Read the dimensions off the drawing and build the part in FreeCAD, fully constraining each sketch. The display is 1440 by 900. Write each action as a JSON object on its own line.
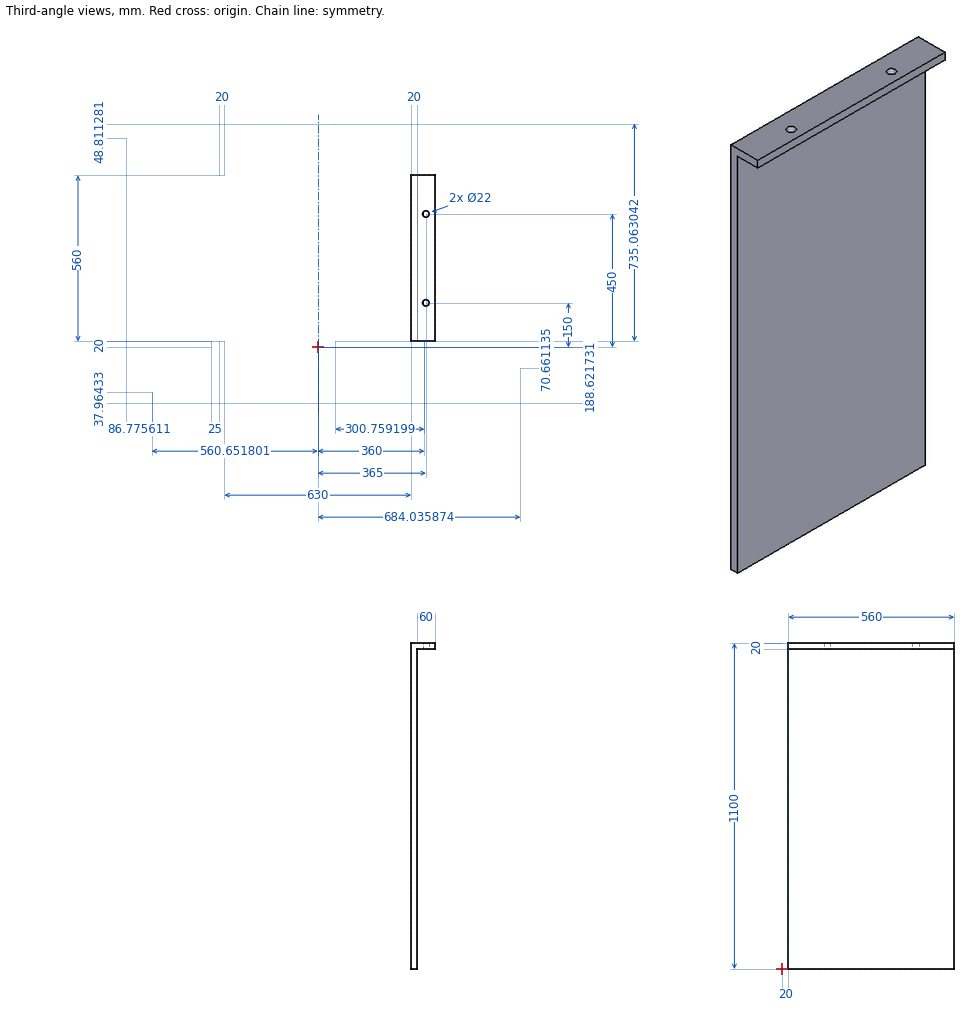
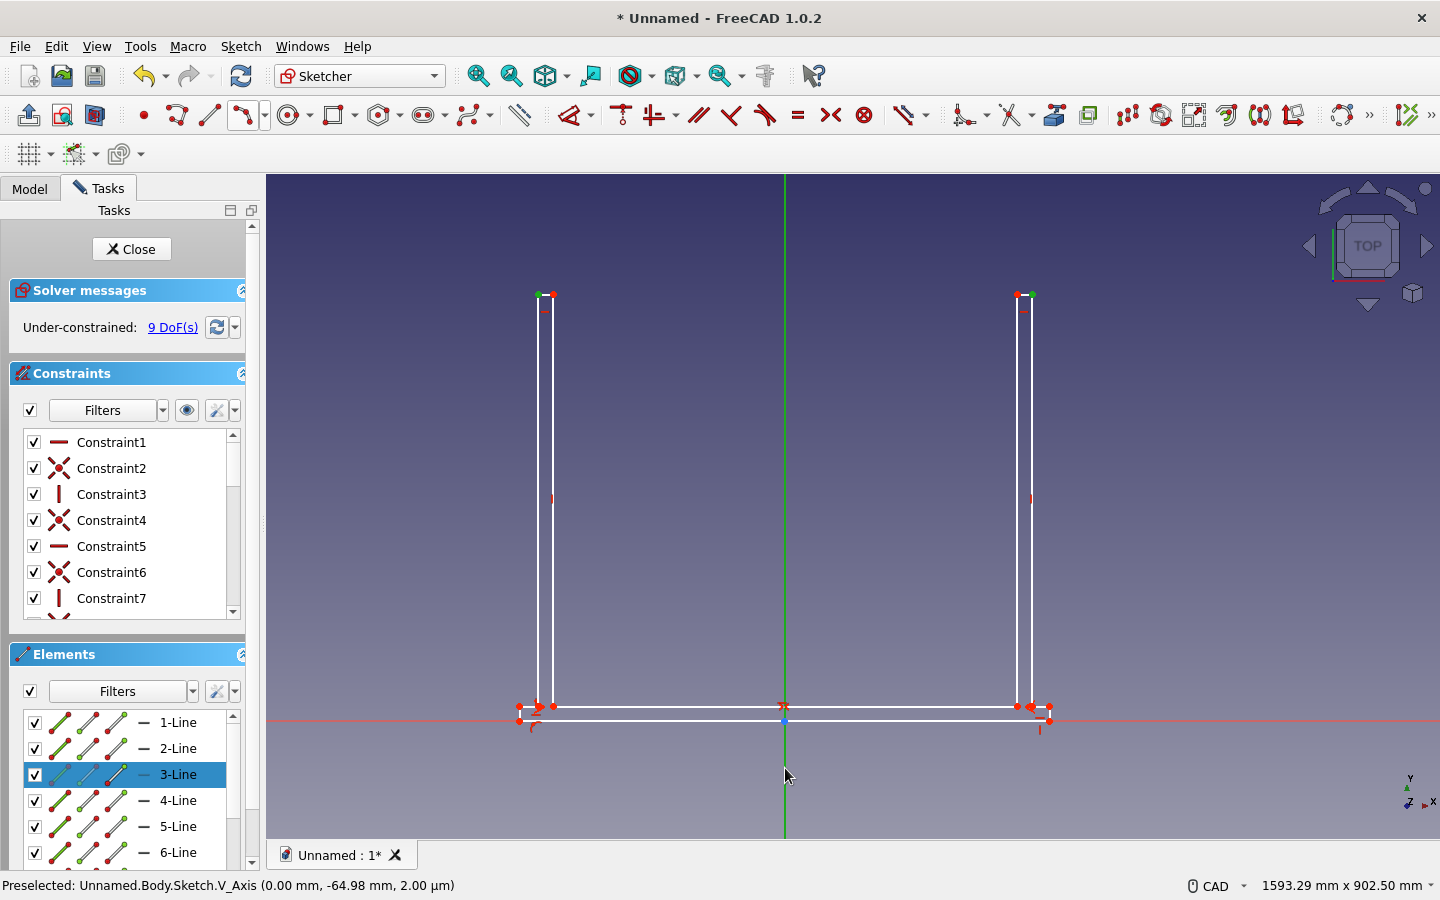
{"action": "key", "text": "s"}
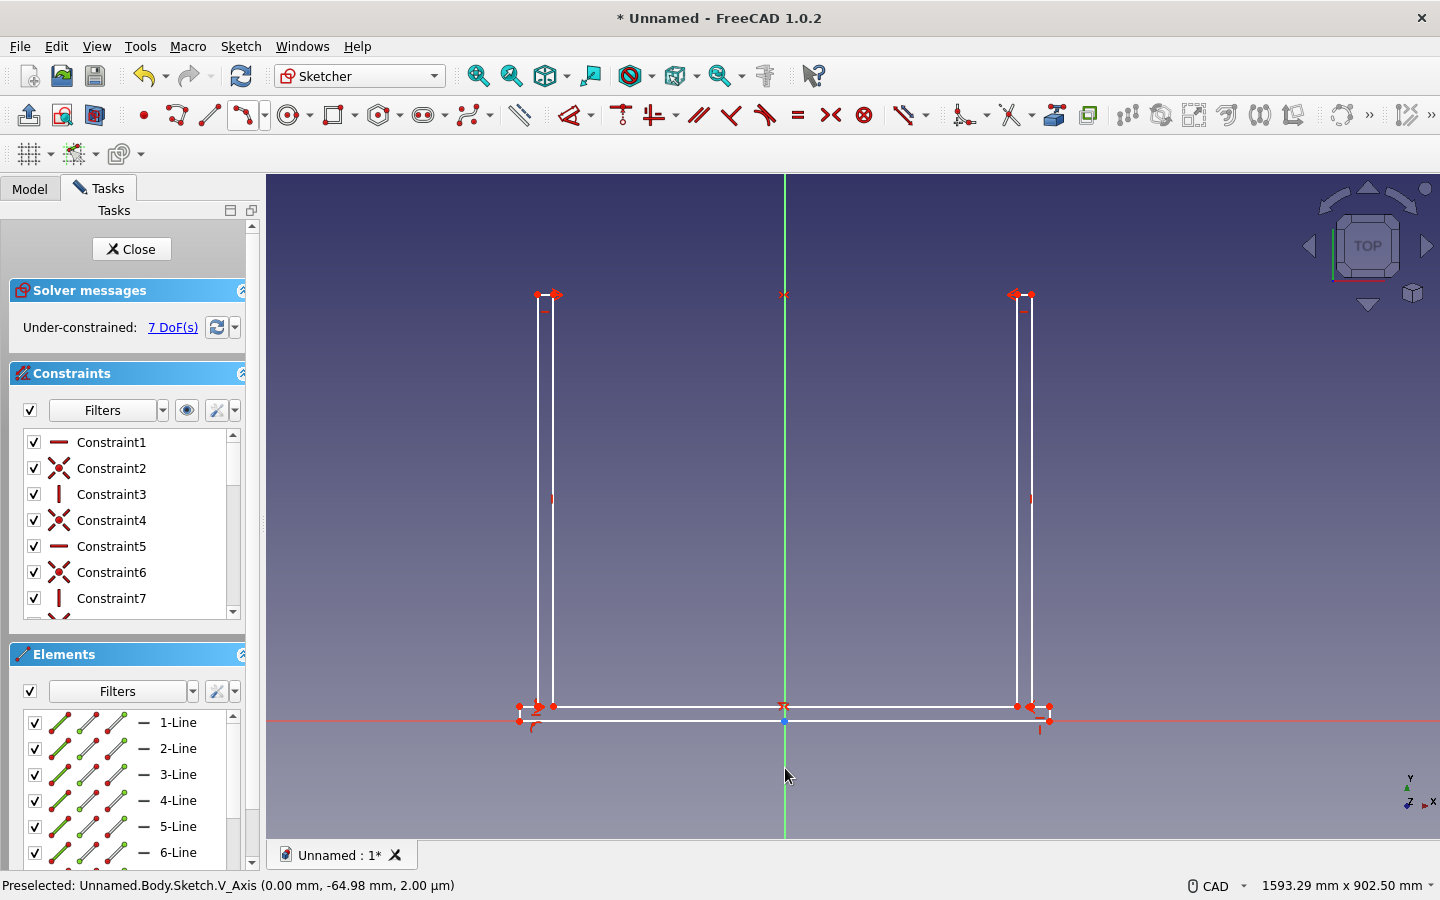
{"action": "left_click", "coordinate": [568, 116]}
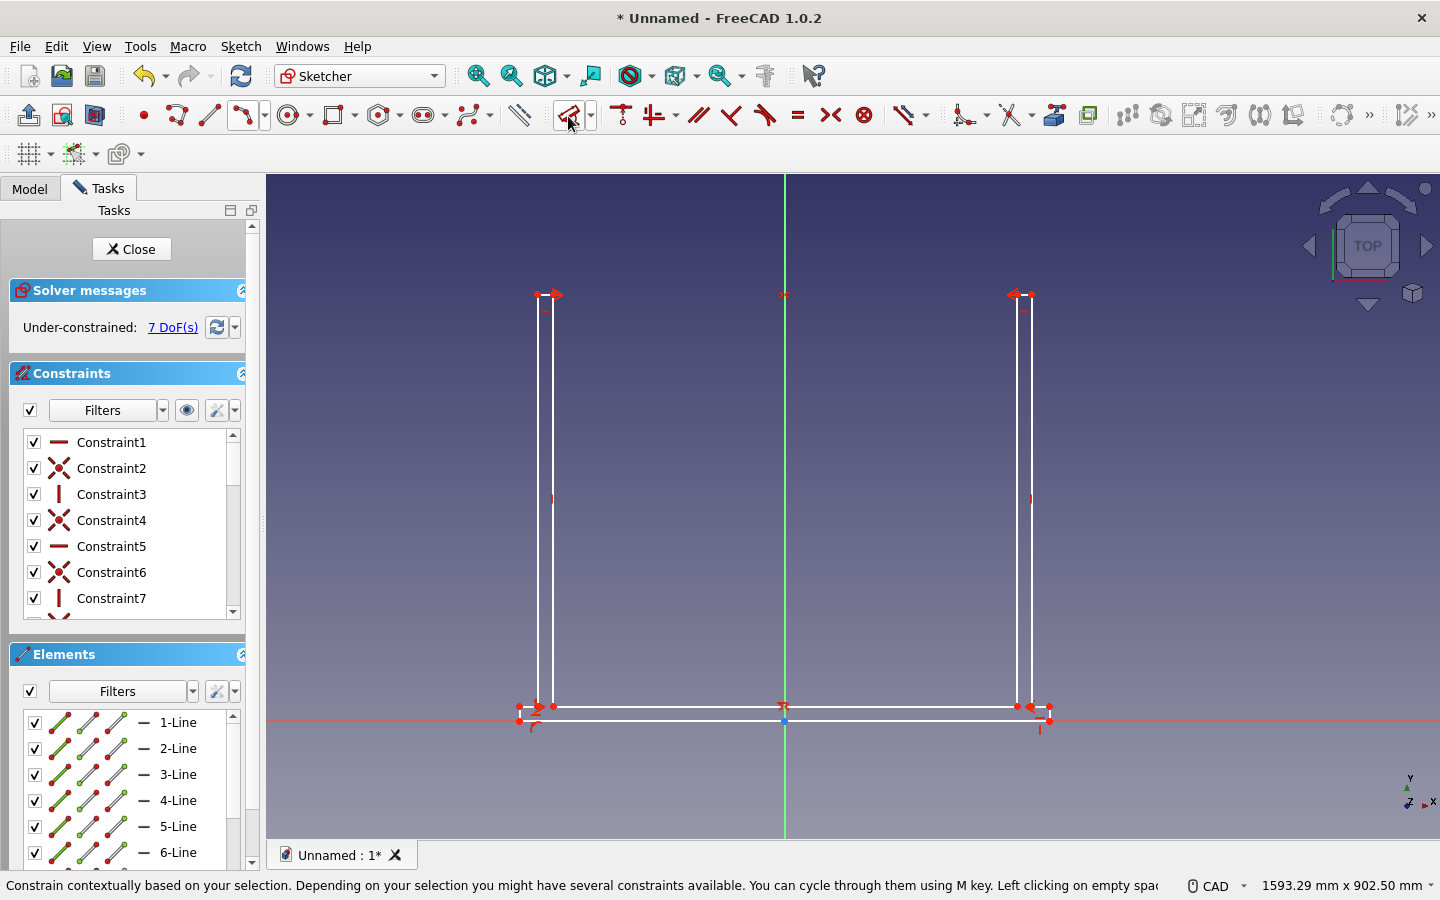
{"action": "scroll", "coordinate": [545, 295], "scroll_direction": "up", "scroll_amount": 5}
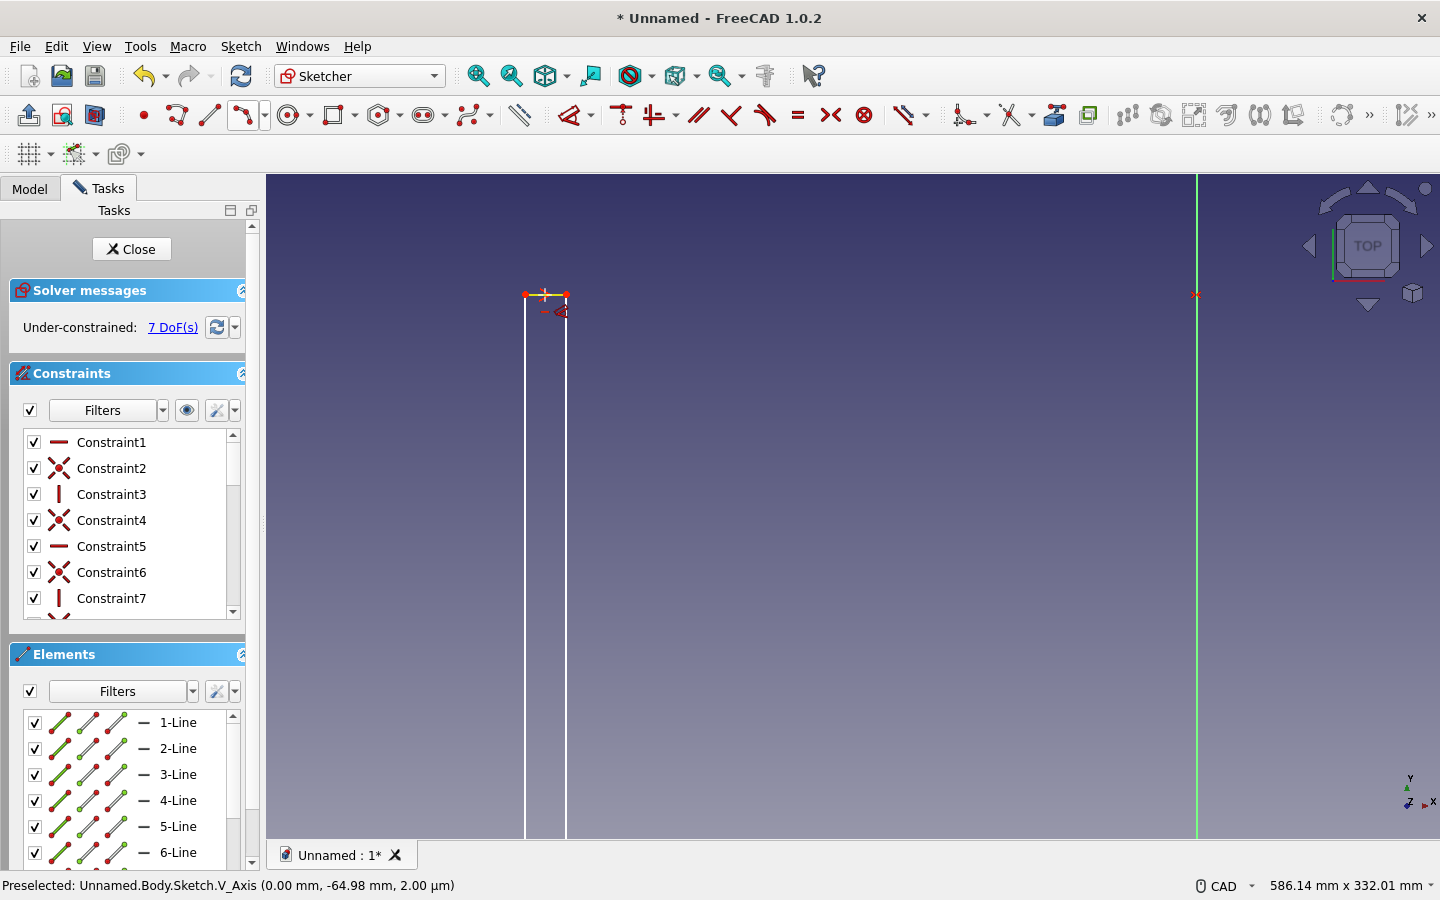
{"action": "left_click", "coordinate": [546, 295]}
{"action": "left_click", "coordinate": [546, 261]}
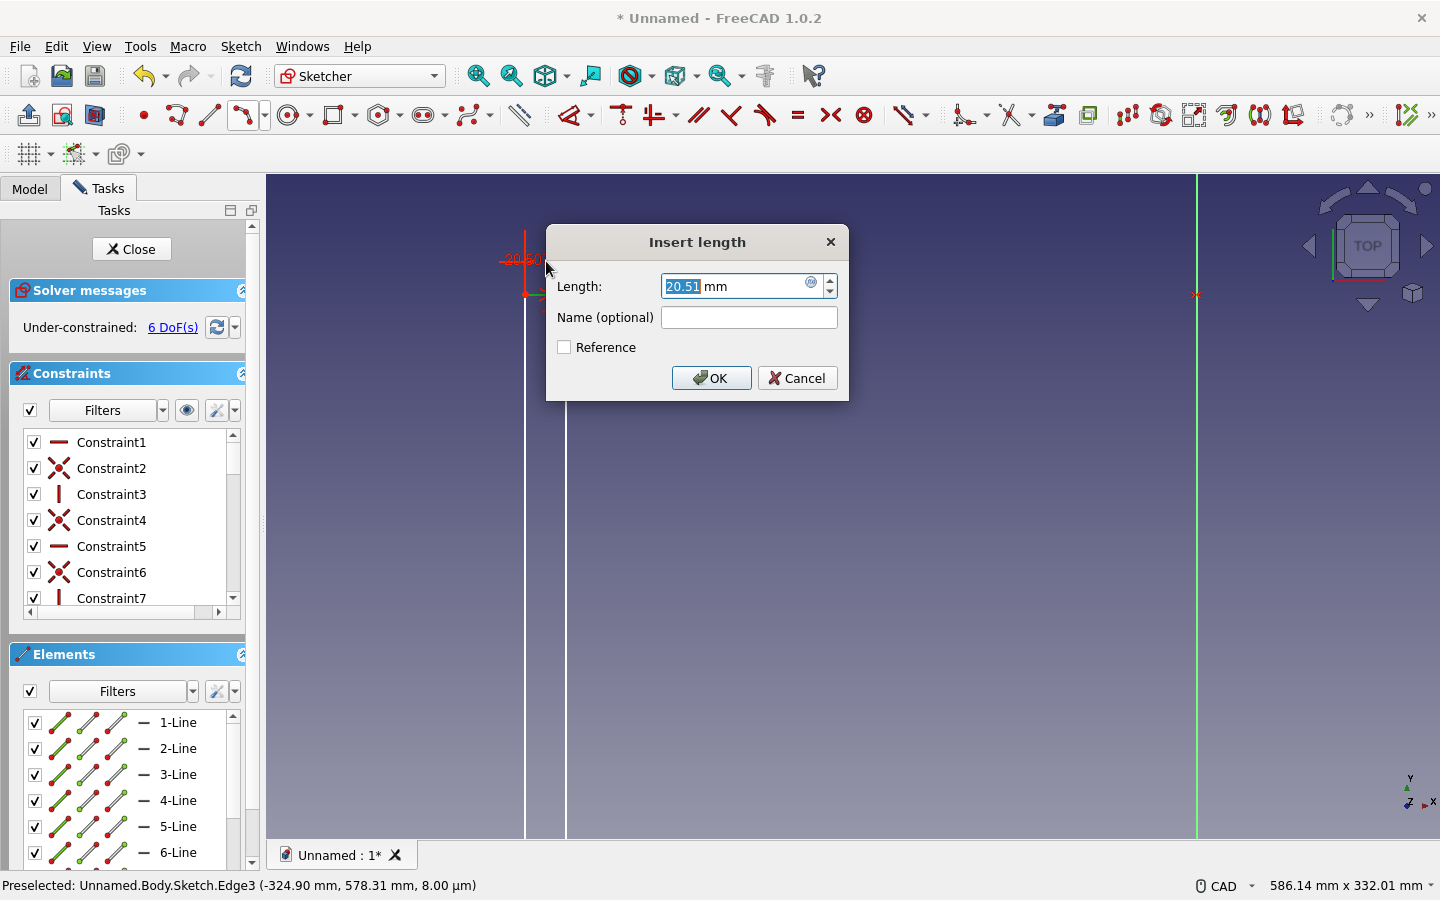
{"action": "type", "text": "20"}
{"action": "key", "text": "Return"}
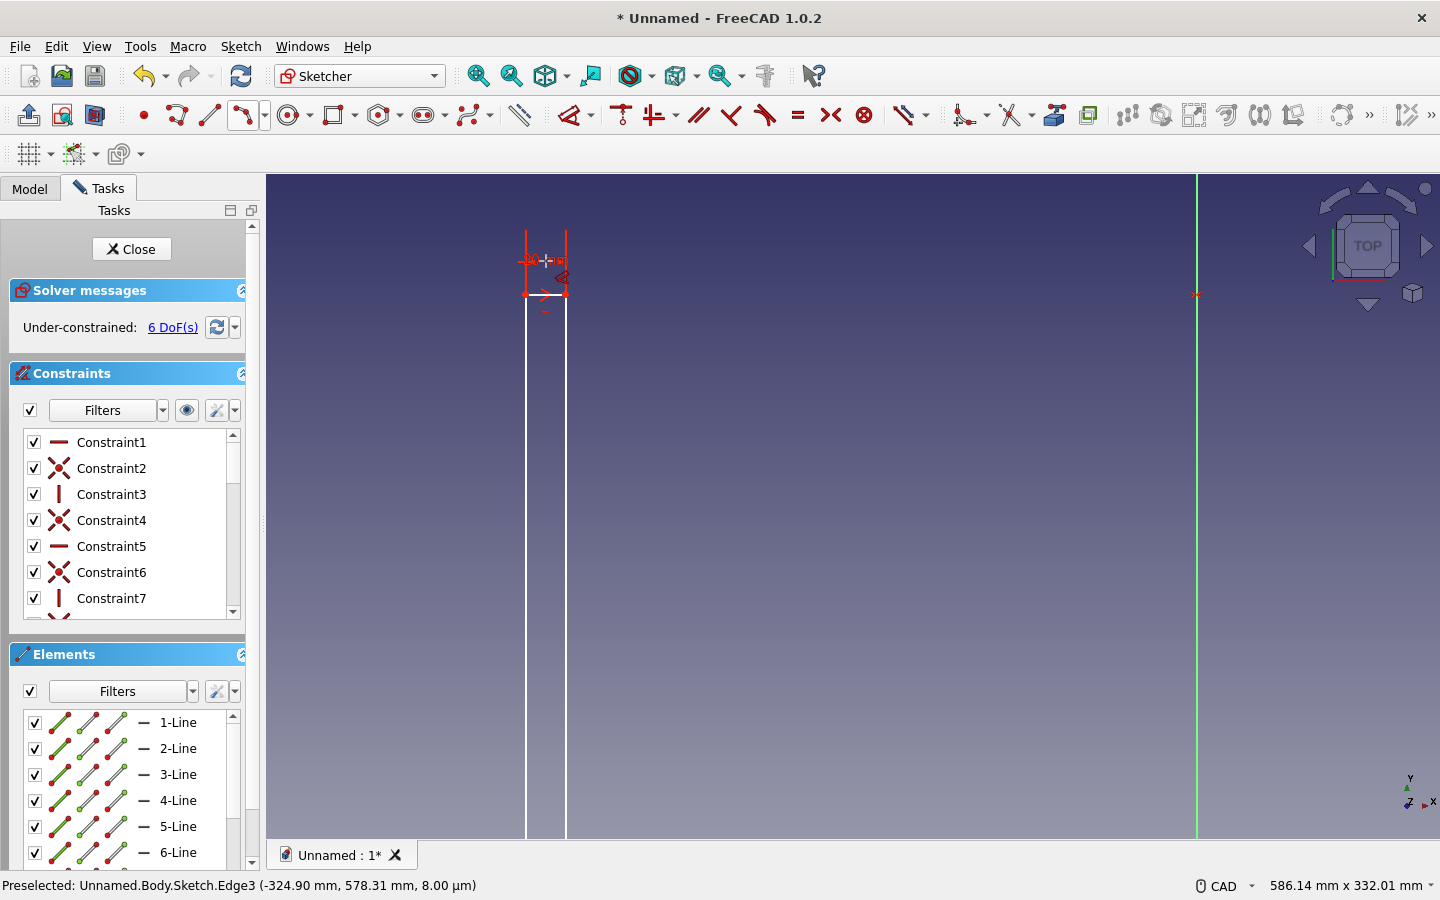
{"action": "scroll", "coordinate": [545, 294], "scroll_direction": "down", "scroll_amount": 5}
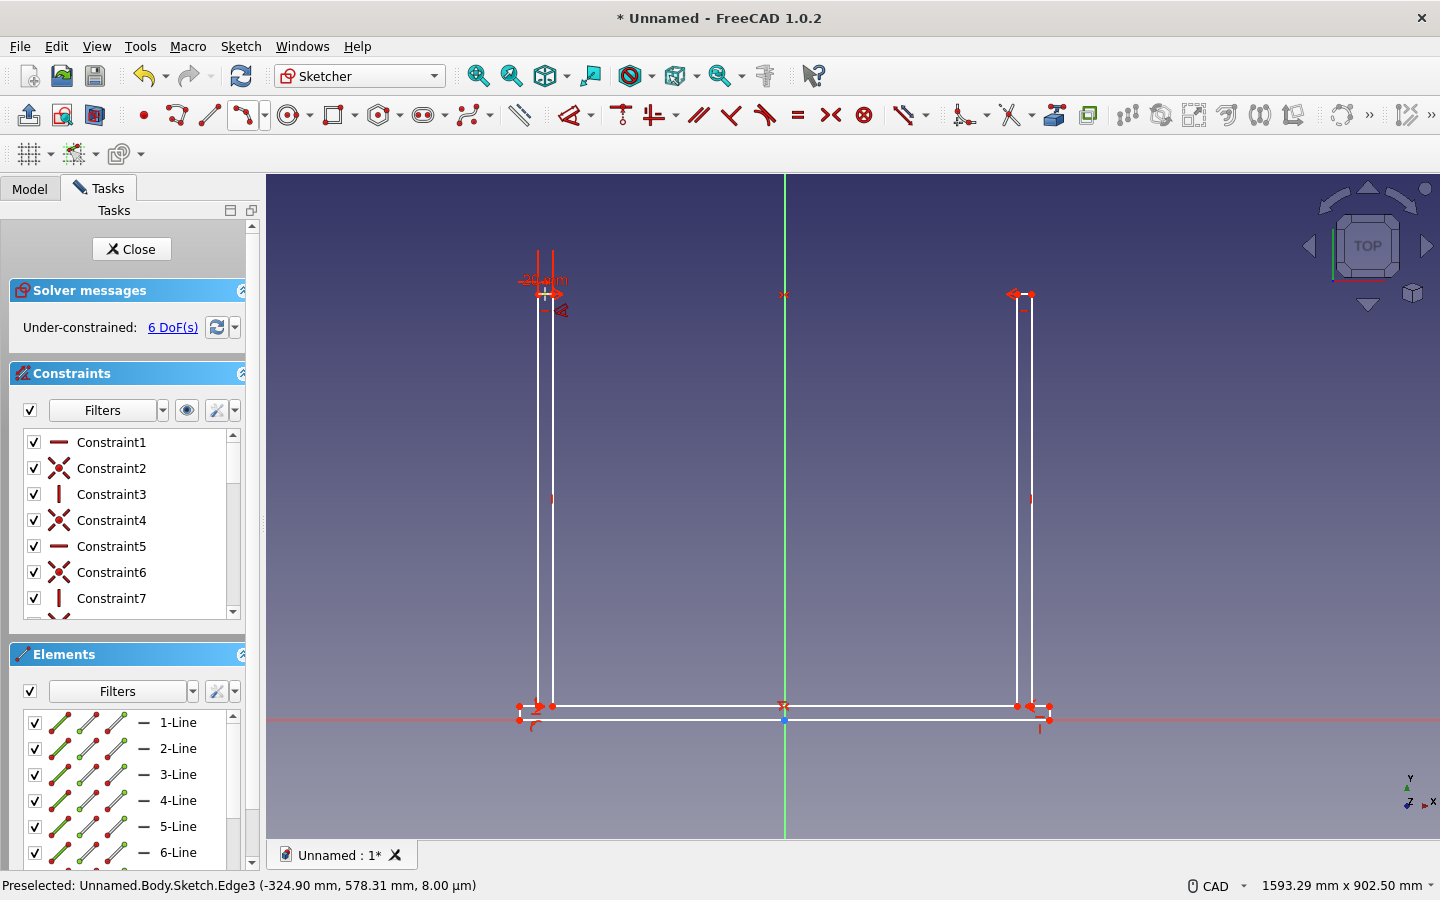
{"action": "scroll", "coordinate": [533, 706], "scroll_direction": "up", "scroll_amount": 5}